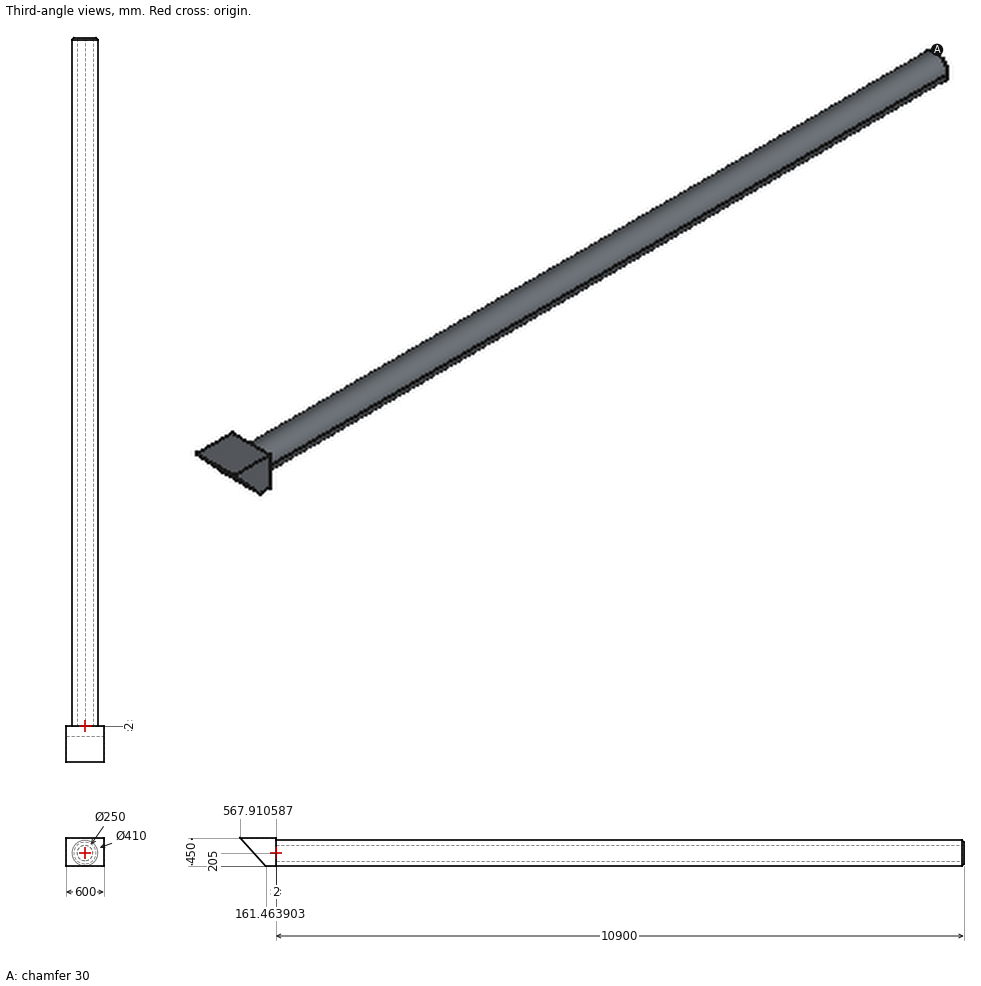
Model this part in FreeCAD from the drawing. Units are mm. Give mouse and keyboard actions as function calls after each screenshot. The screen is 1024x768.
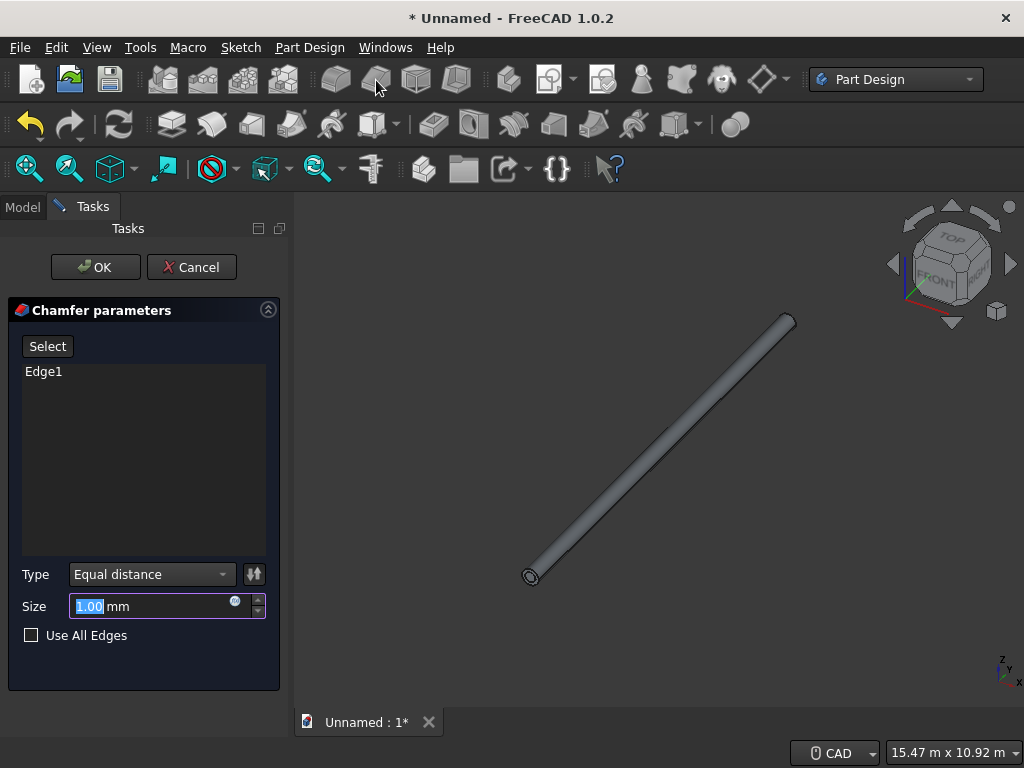
text(30)
key(Tab)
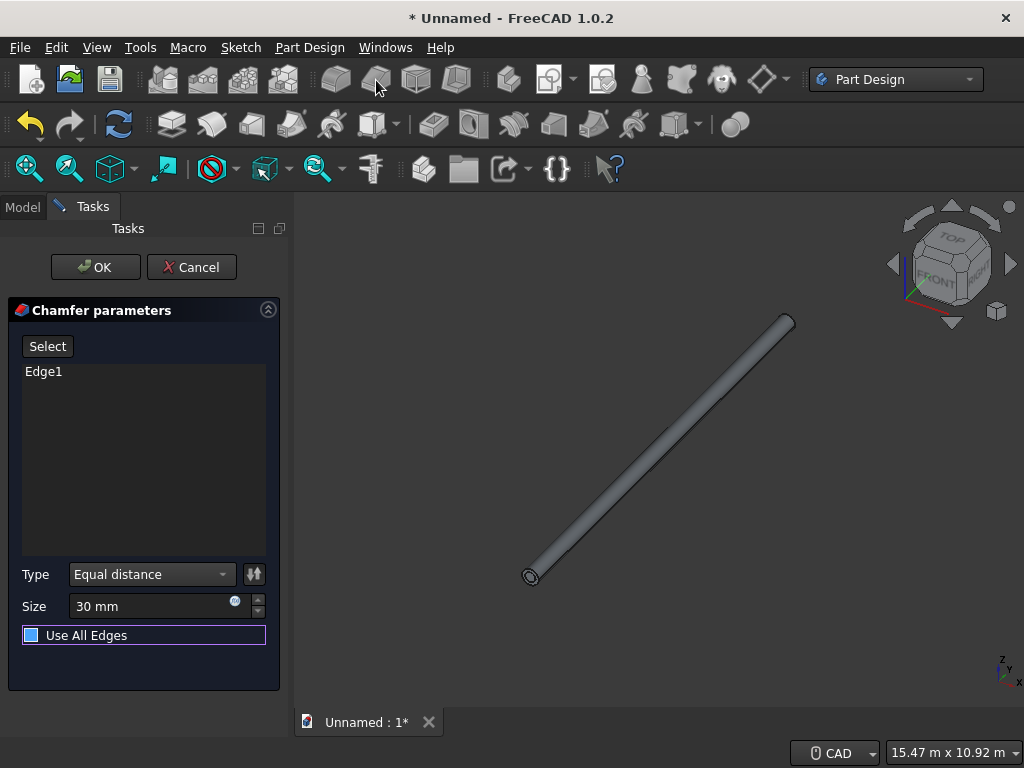
click(96, 267)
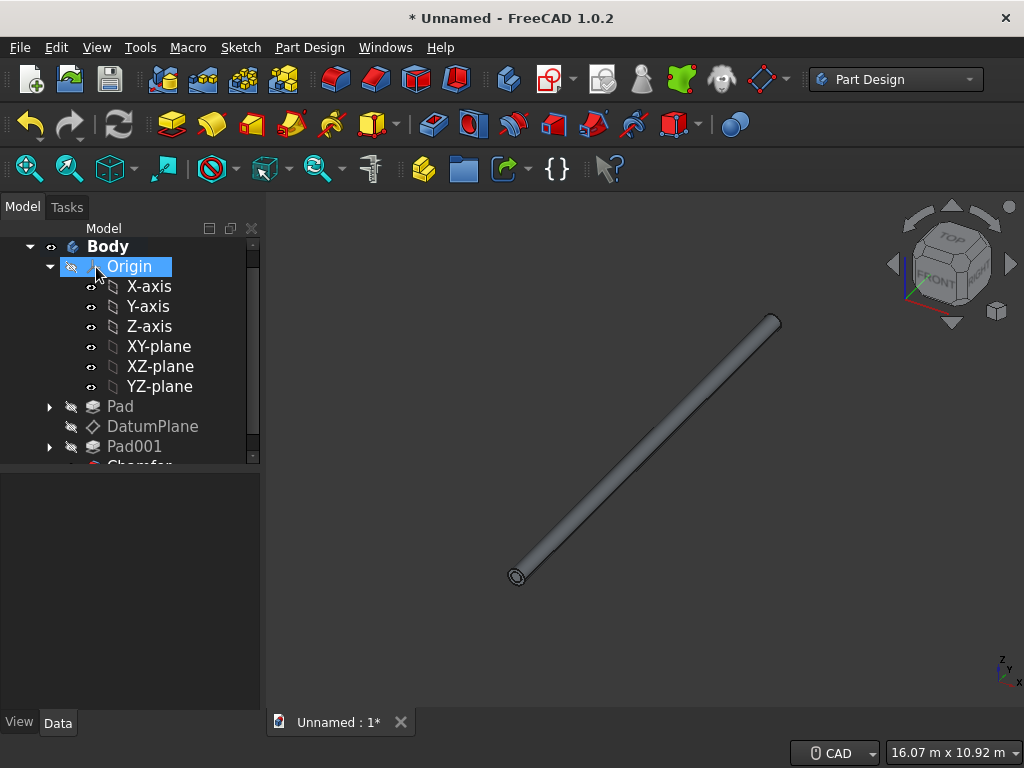
click(550, 80)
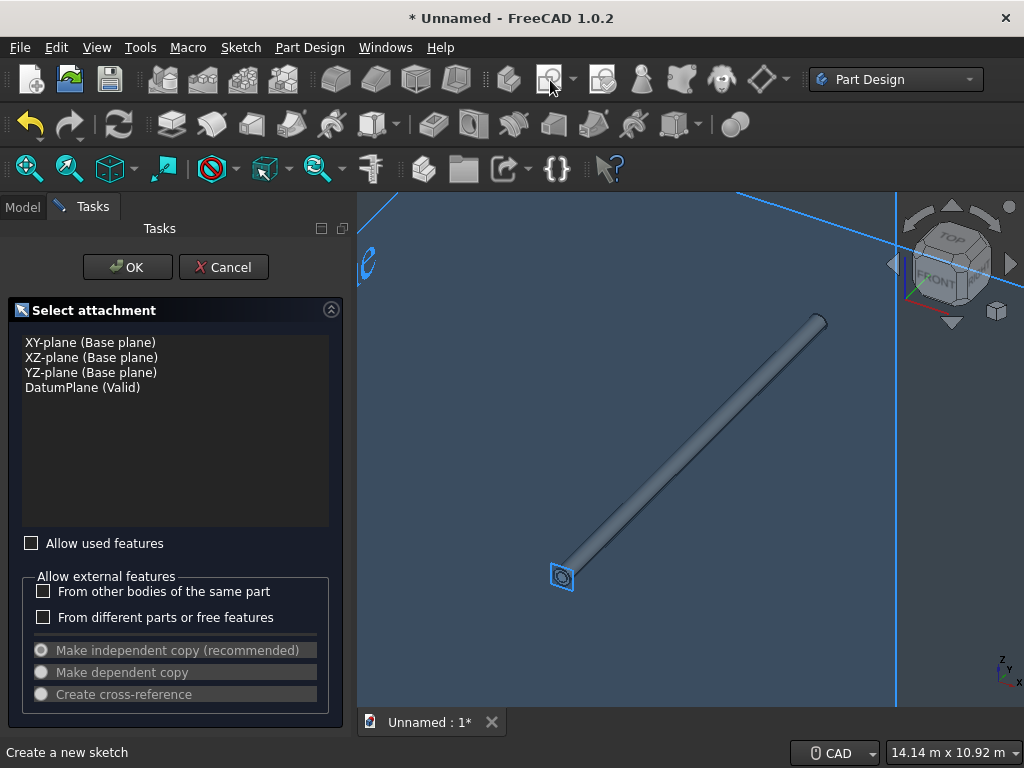
click(82, 372)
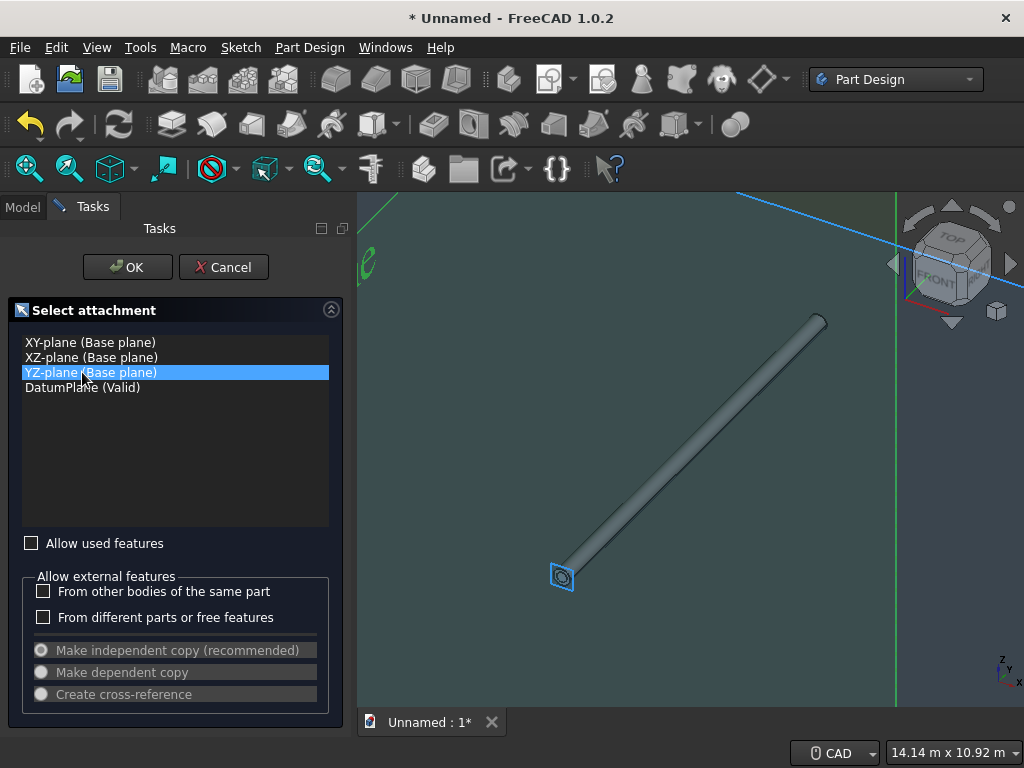
click(128, 267)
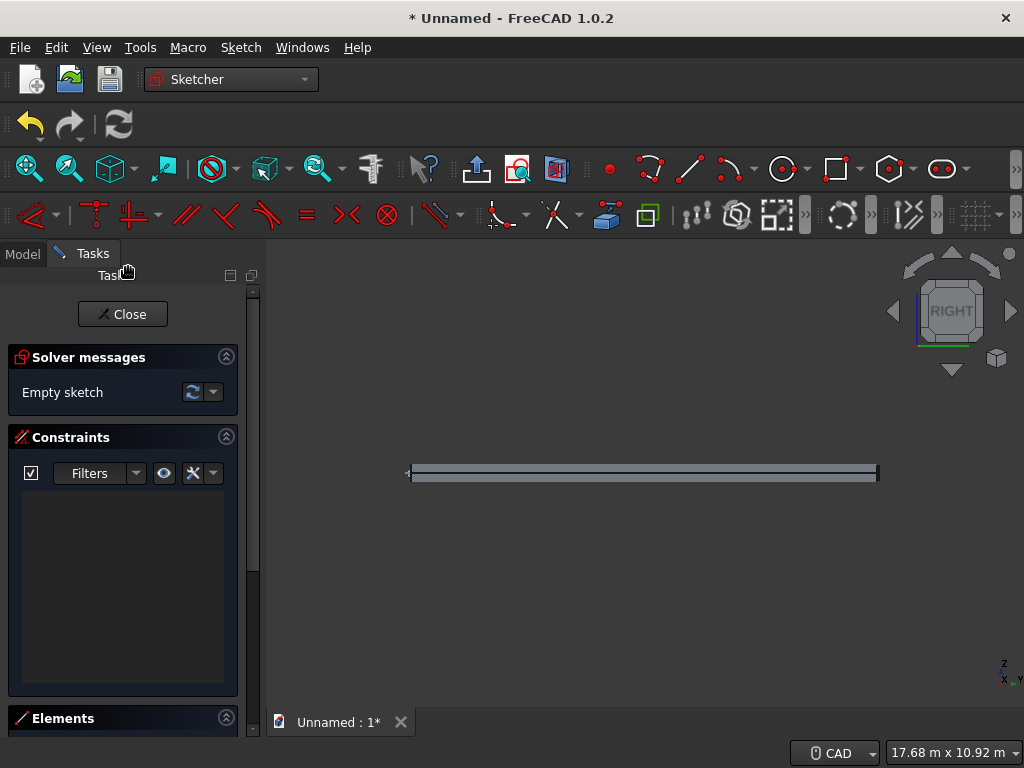
click(558, 170)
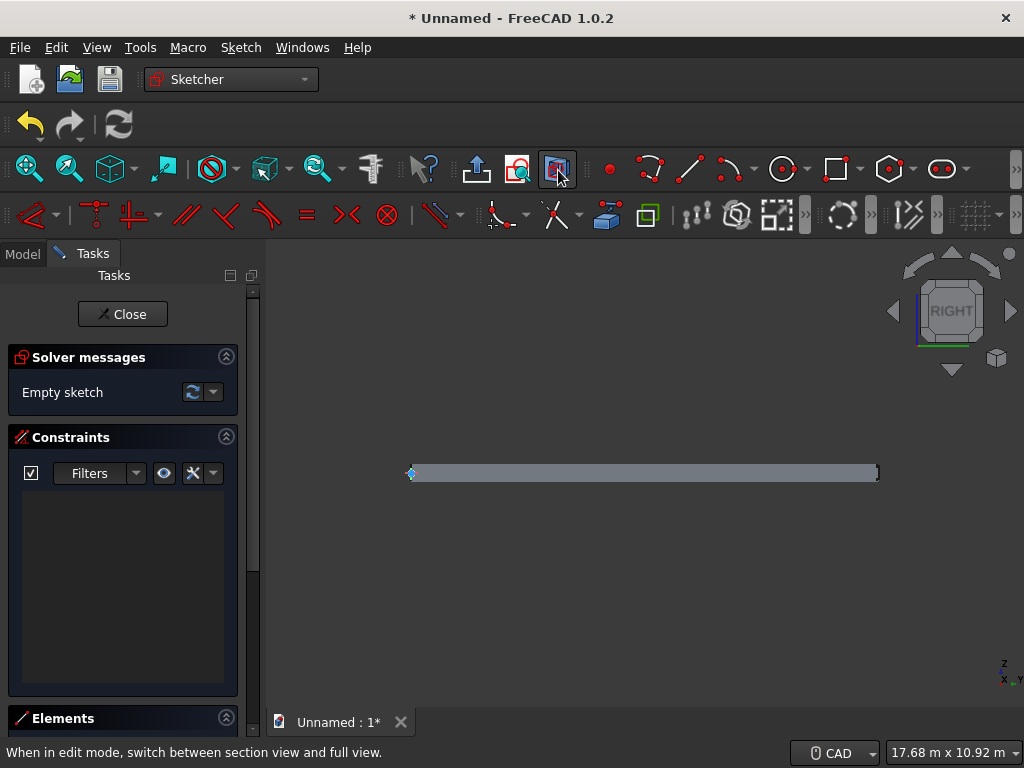
scroll(388, 472, up, 14)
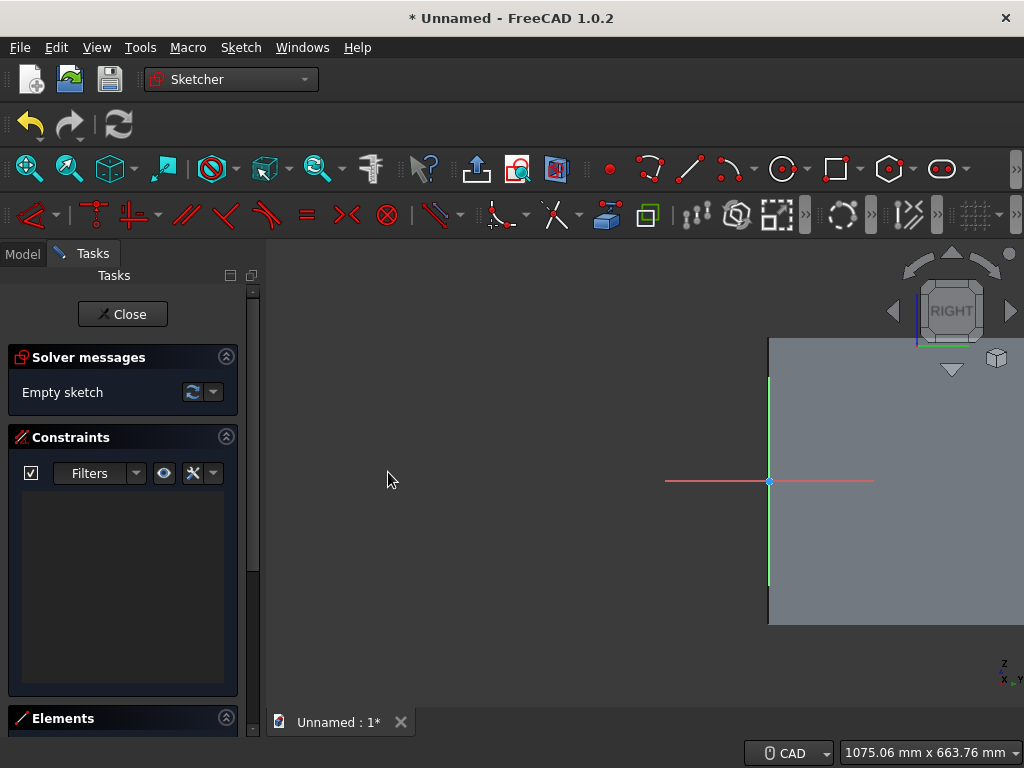
click(650, 170)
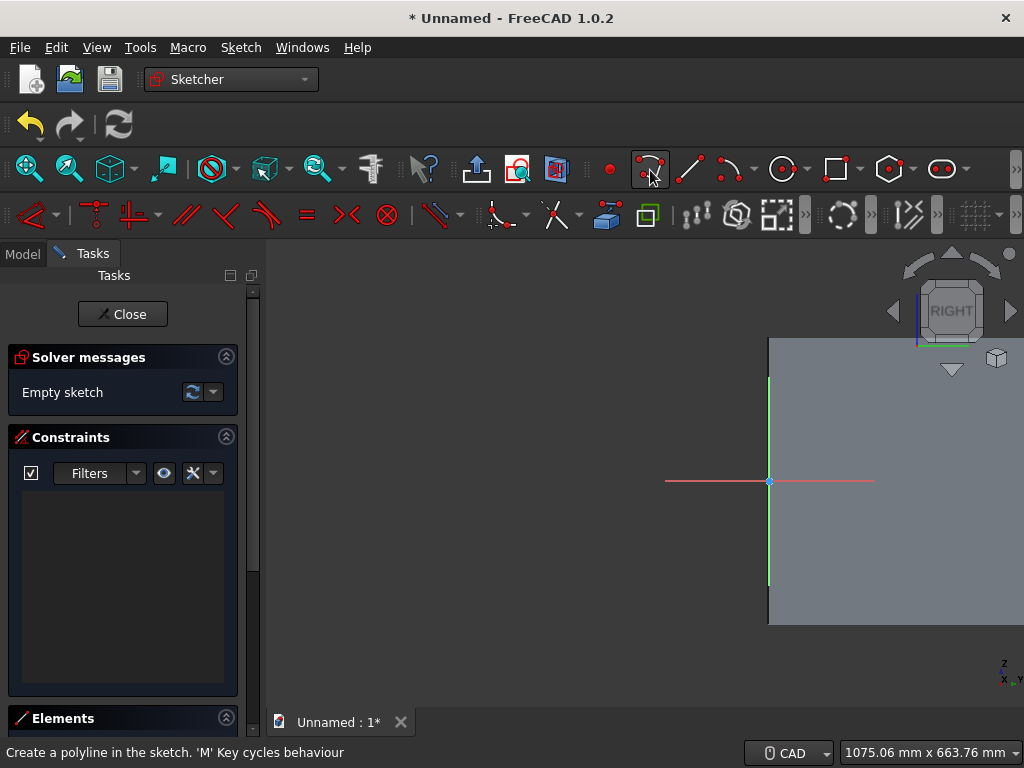
scroll(768, 626, up, 13)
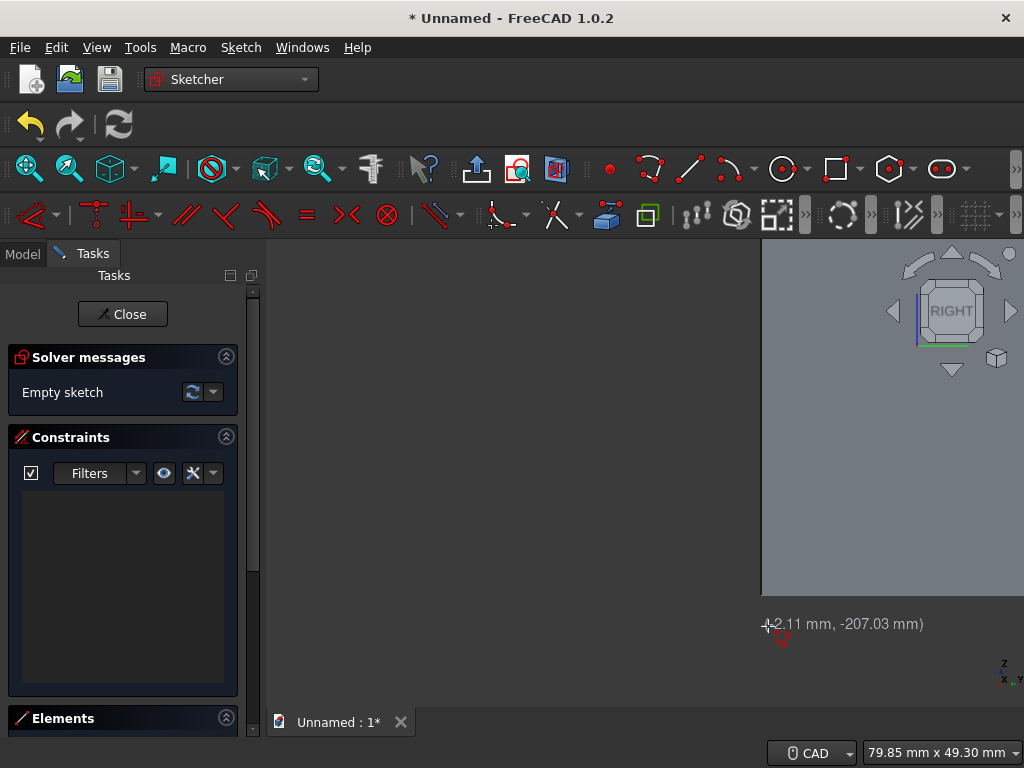
click(761, 610)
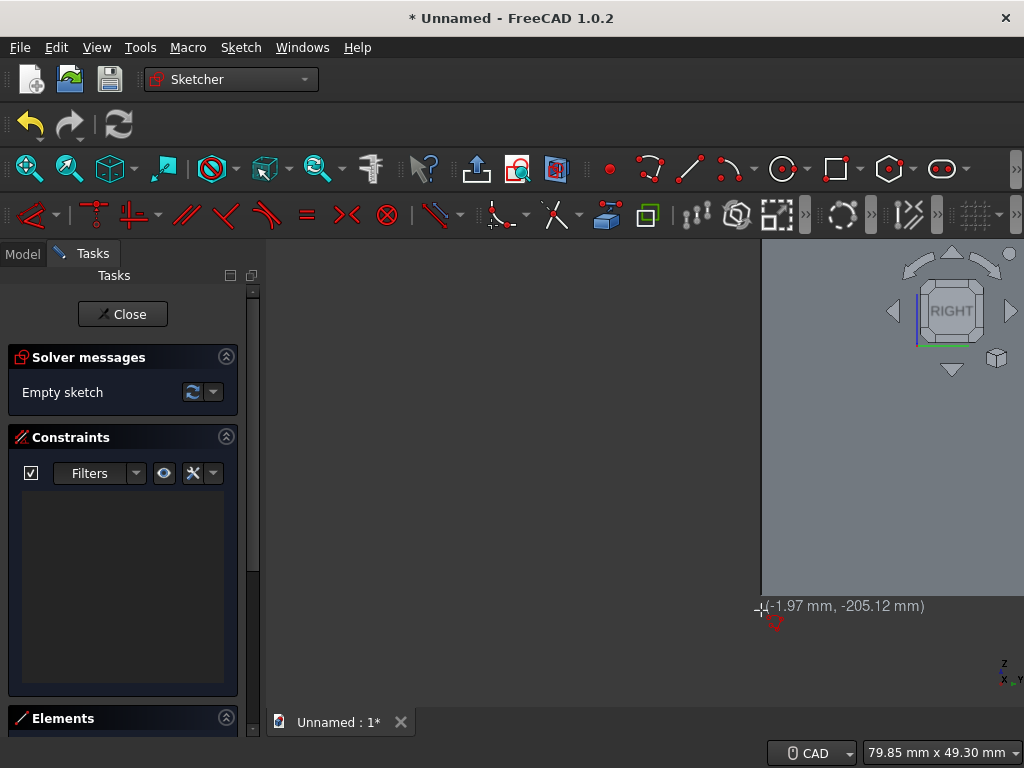
scroll(777, 633, down, 13)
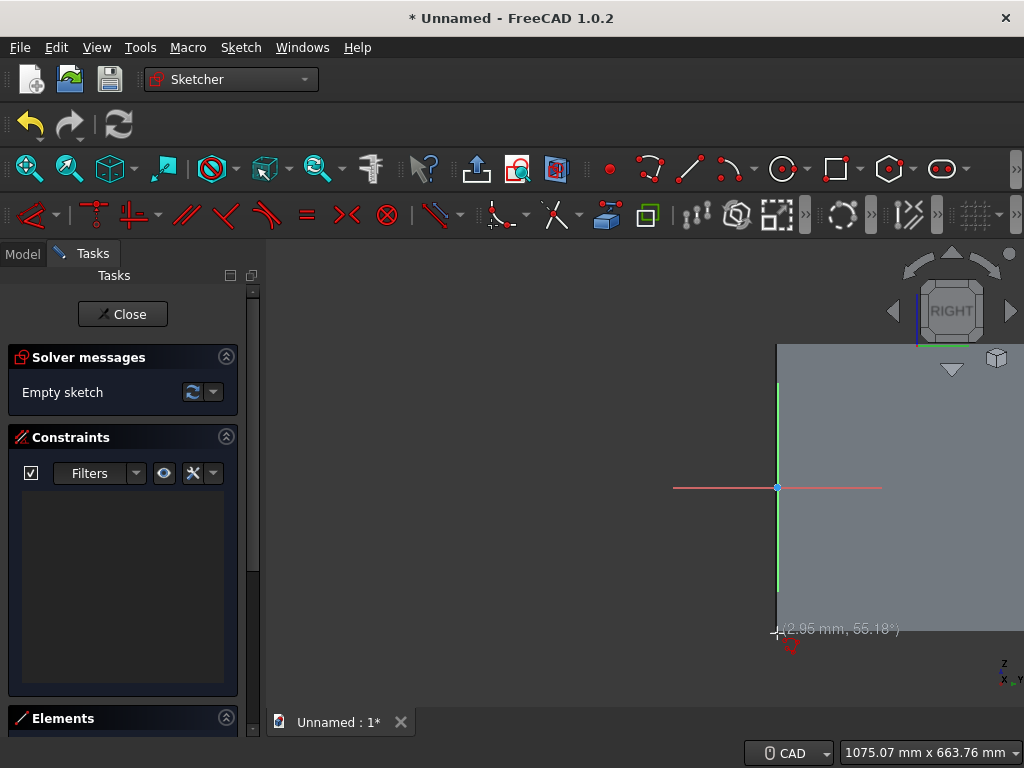
scroll(776, 315, up, 13)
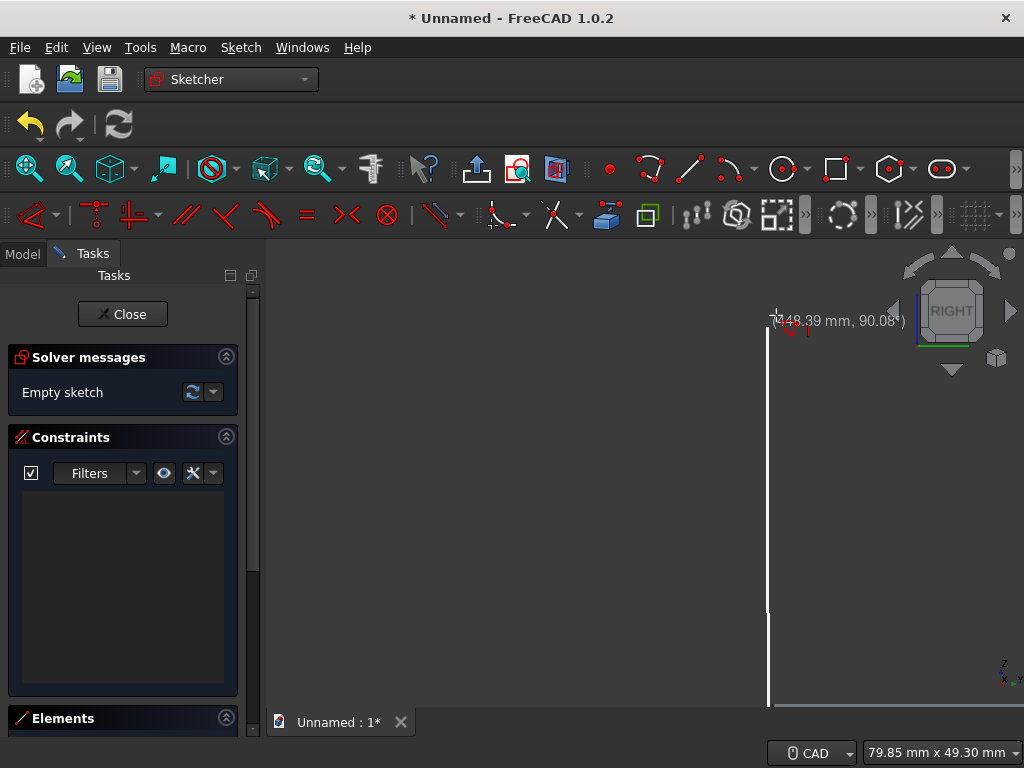
click(773, 310)